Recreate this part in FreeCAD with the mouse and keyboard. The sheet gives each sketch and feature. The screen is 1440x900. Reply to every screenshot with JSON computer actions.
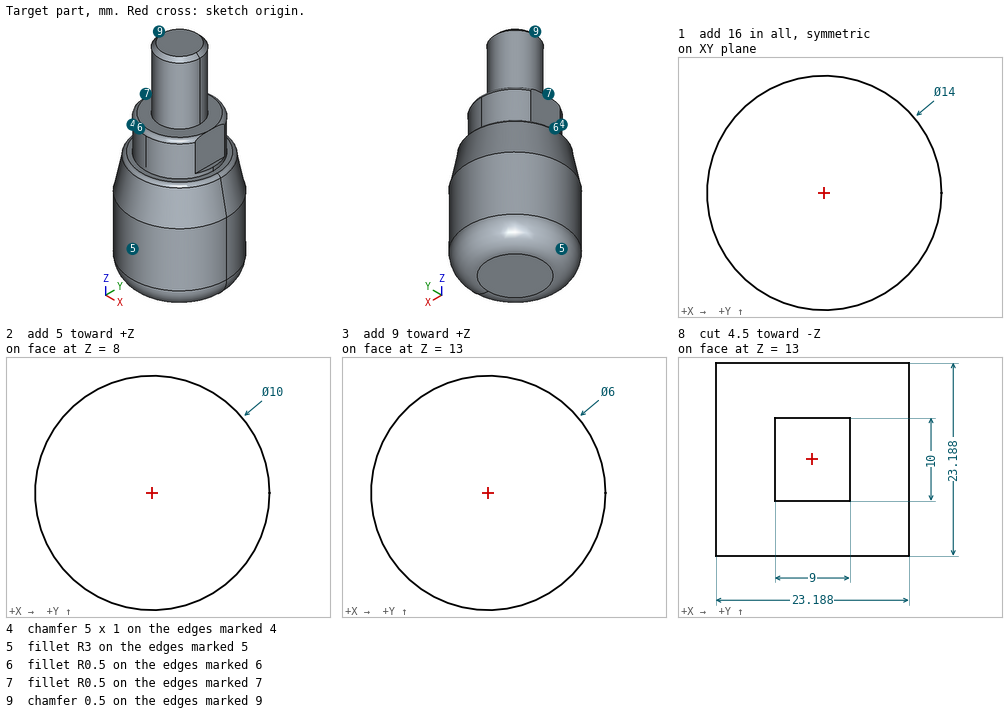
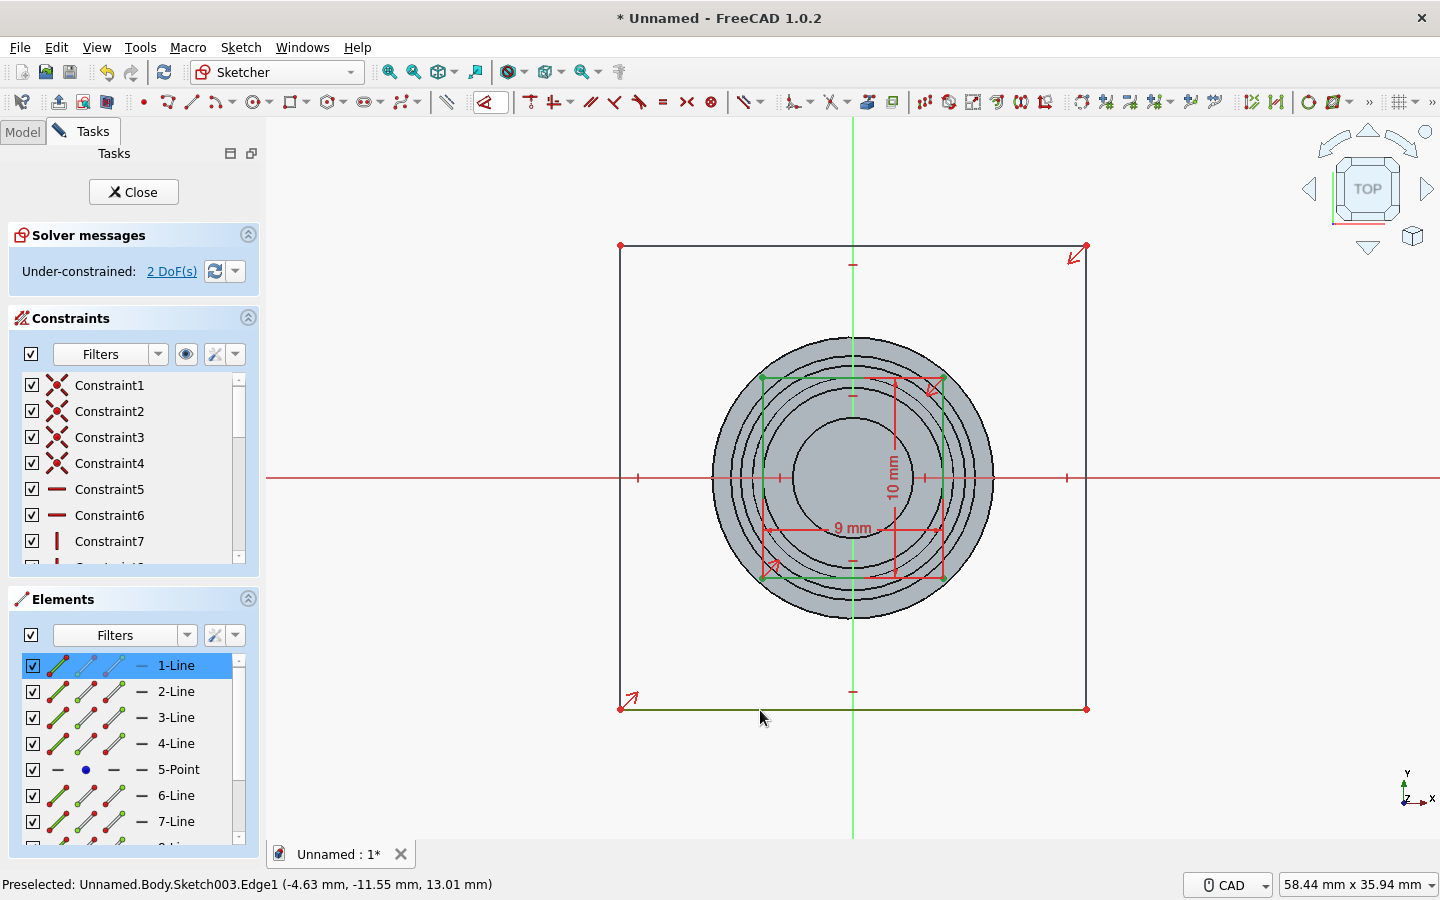
{"action": "key", "text": "l"}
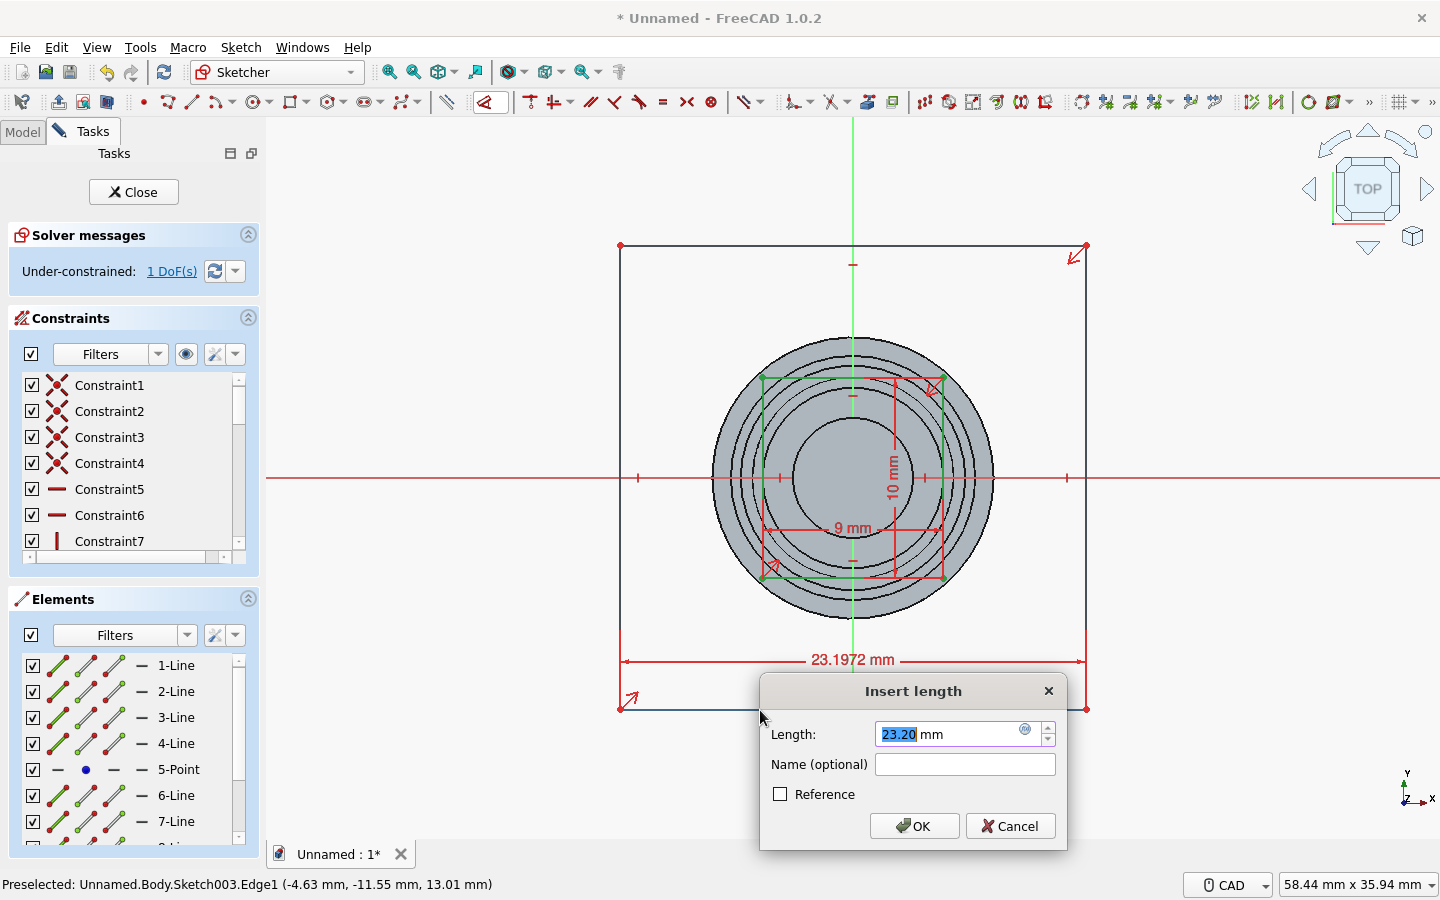
{"action": "type", "text": "23.188"}
{"action": "key", "text": "Return"}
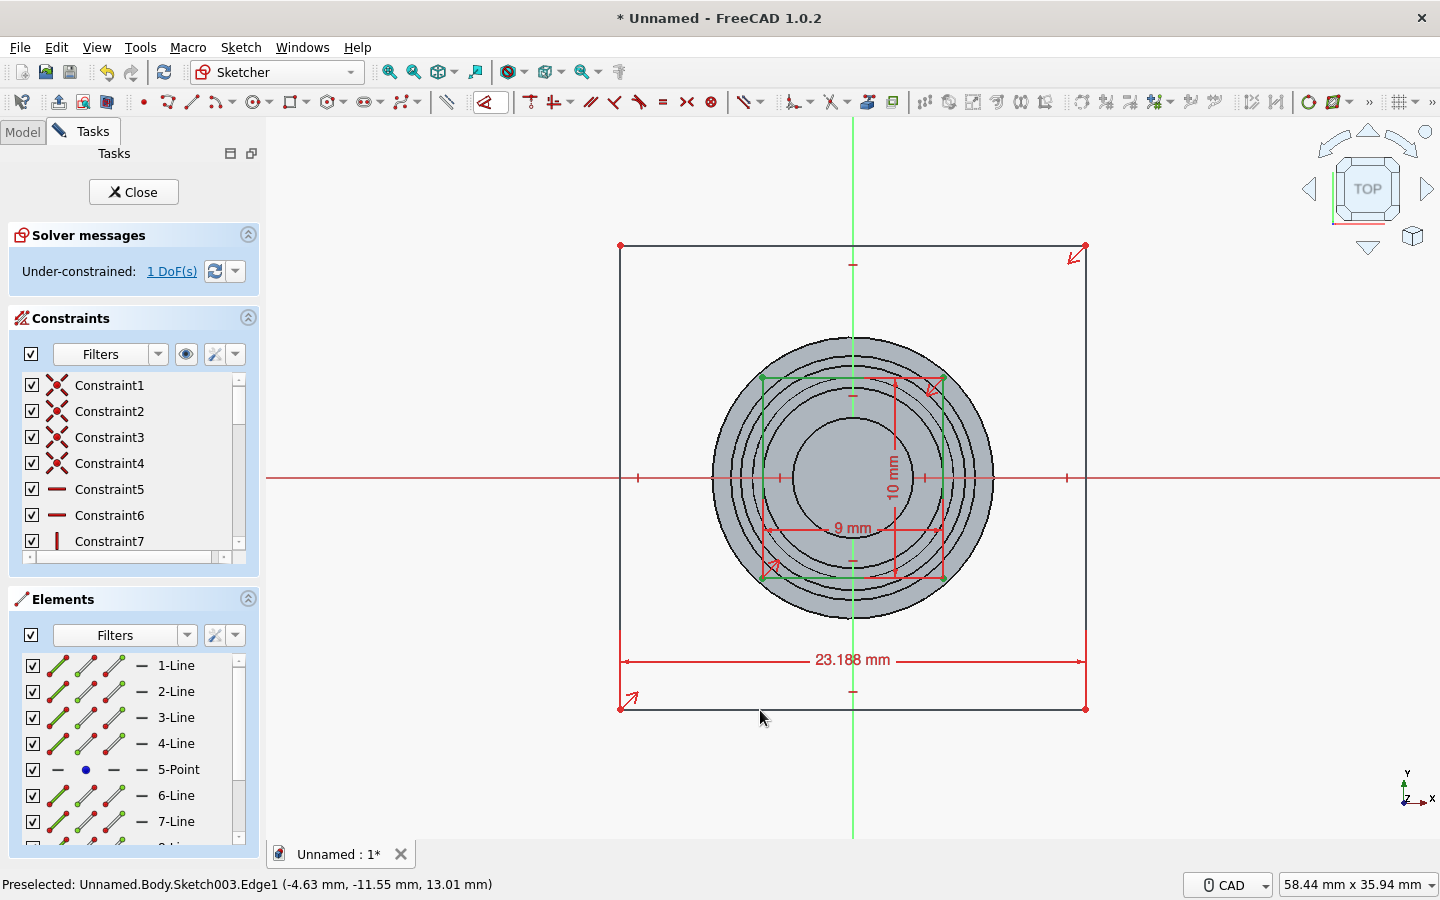
{"action": "left_click", "coordinate": [1086, 571]}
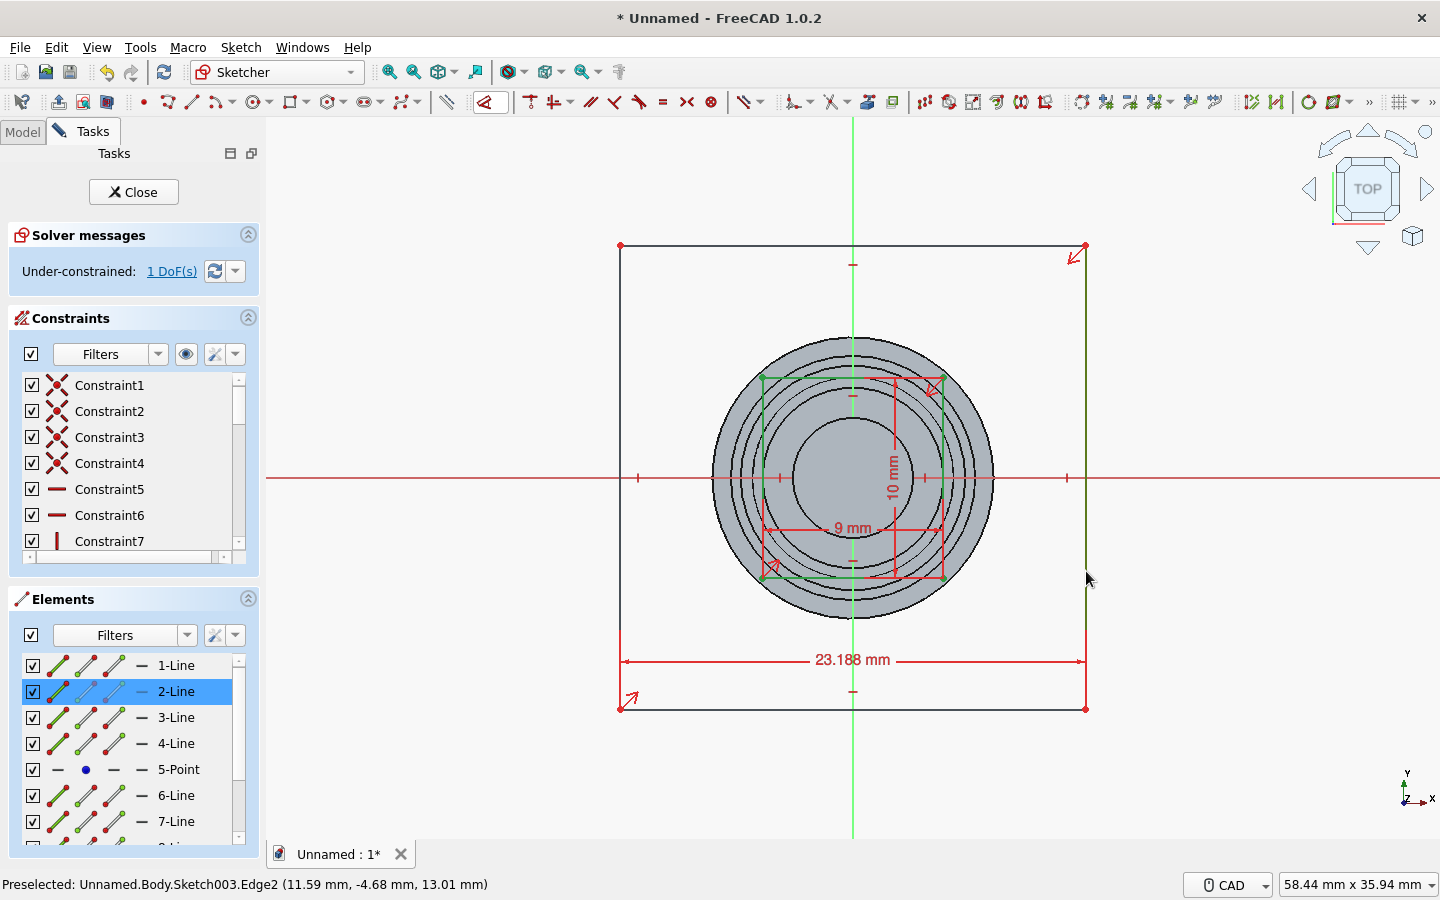
{"action": "key", "text": "i"}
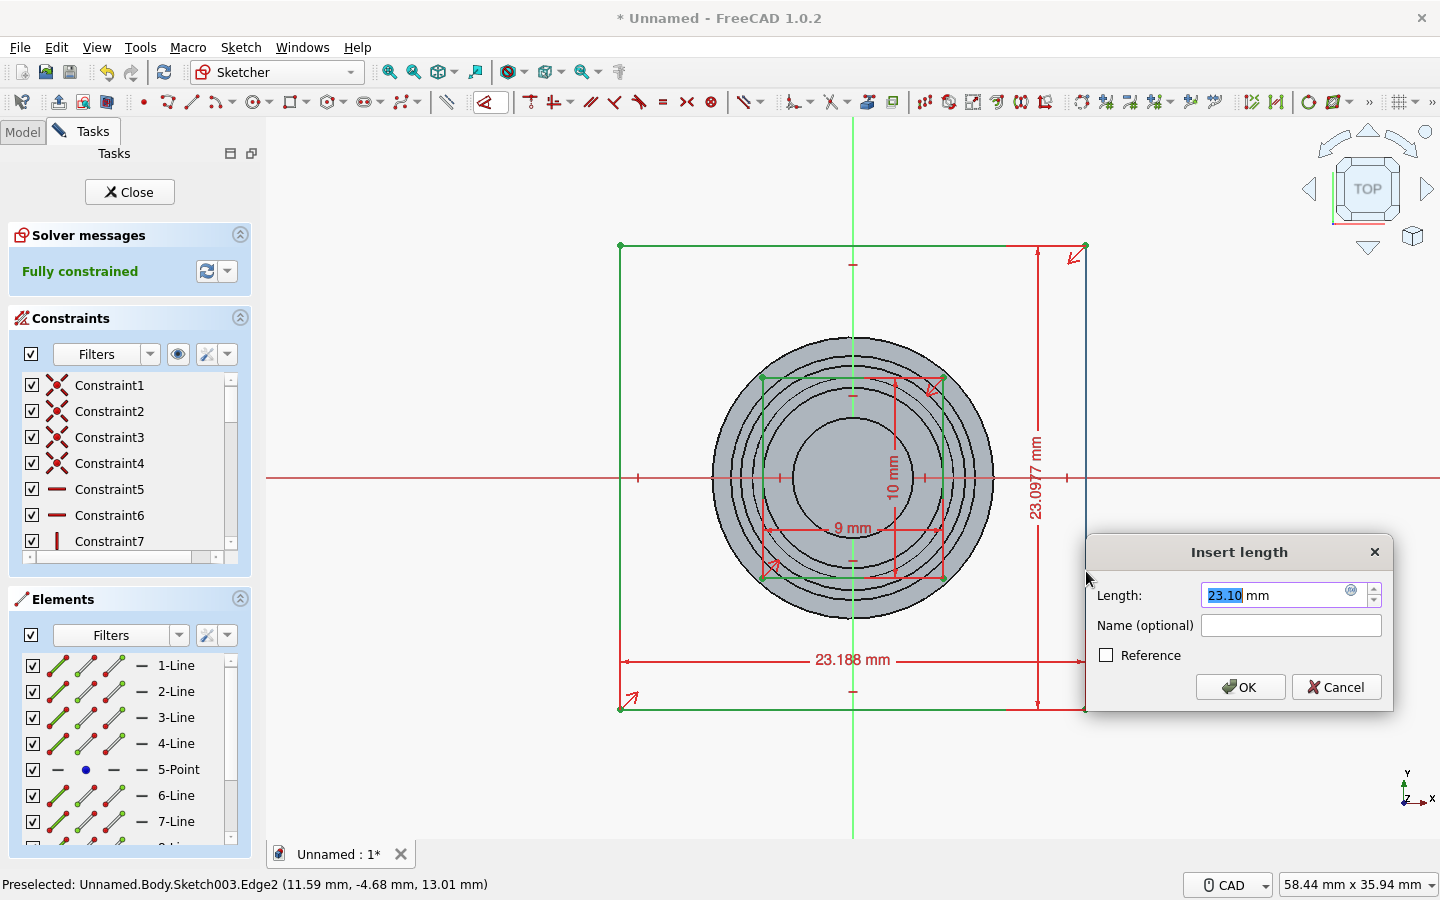
{"action": "type", "text": "23.188"}
{"action": "key", "text": "Return"}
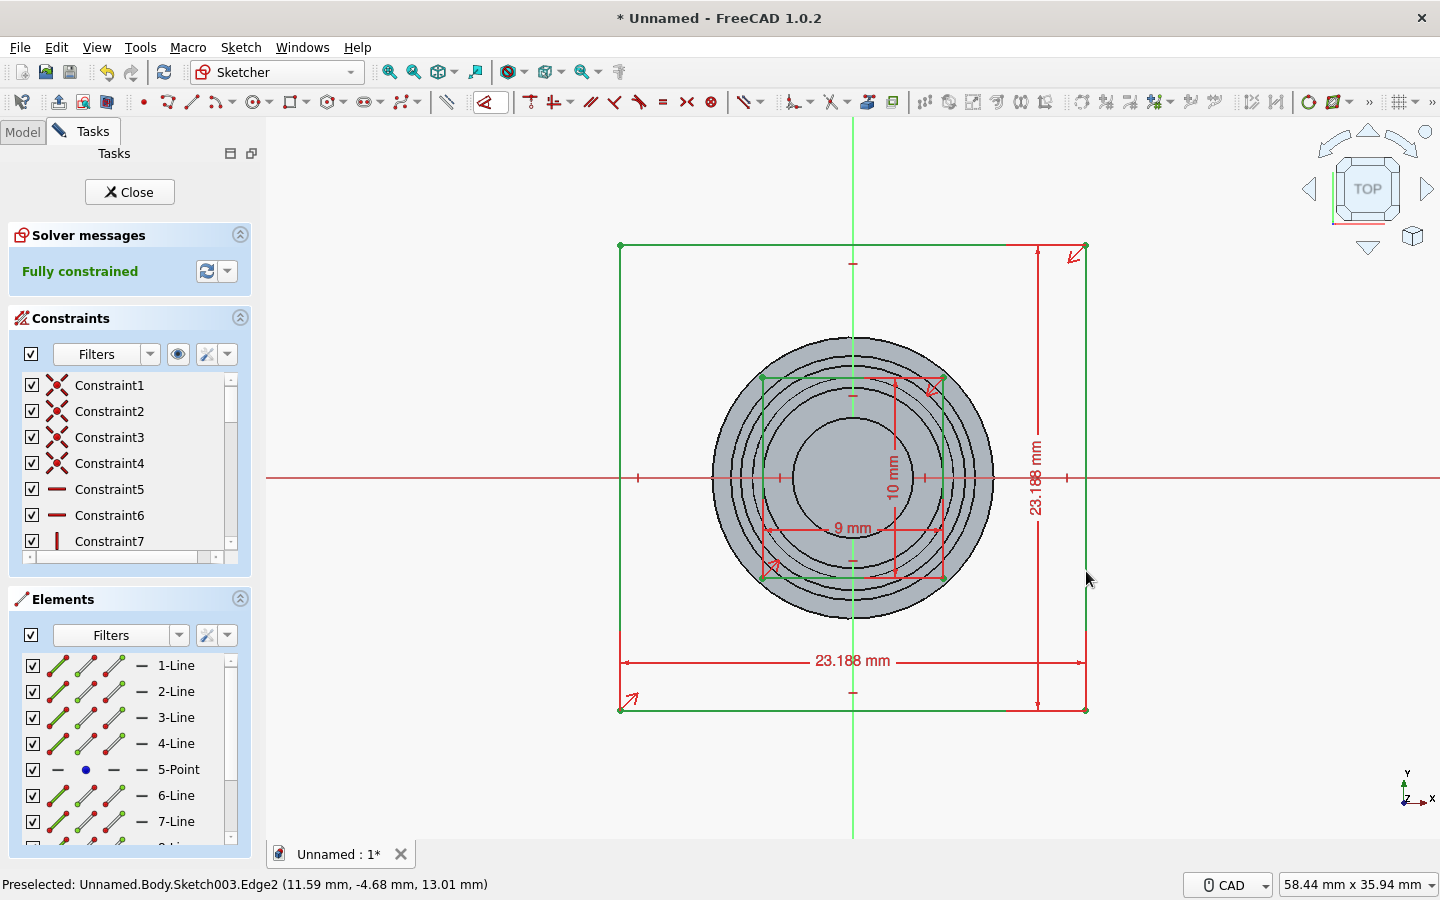
{"action": "left_click", "coordinate": [130, 192]}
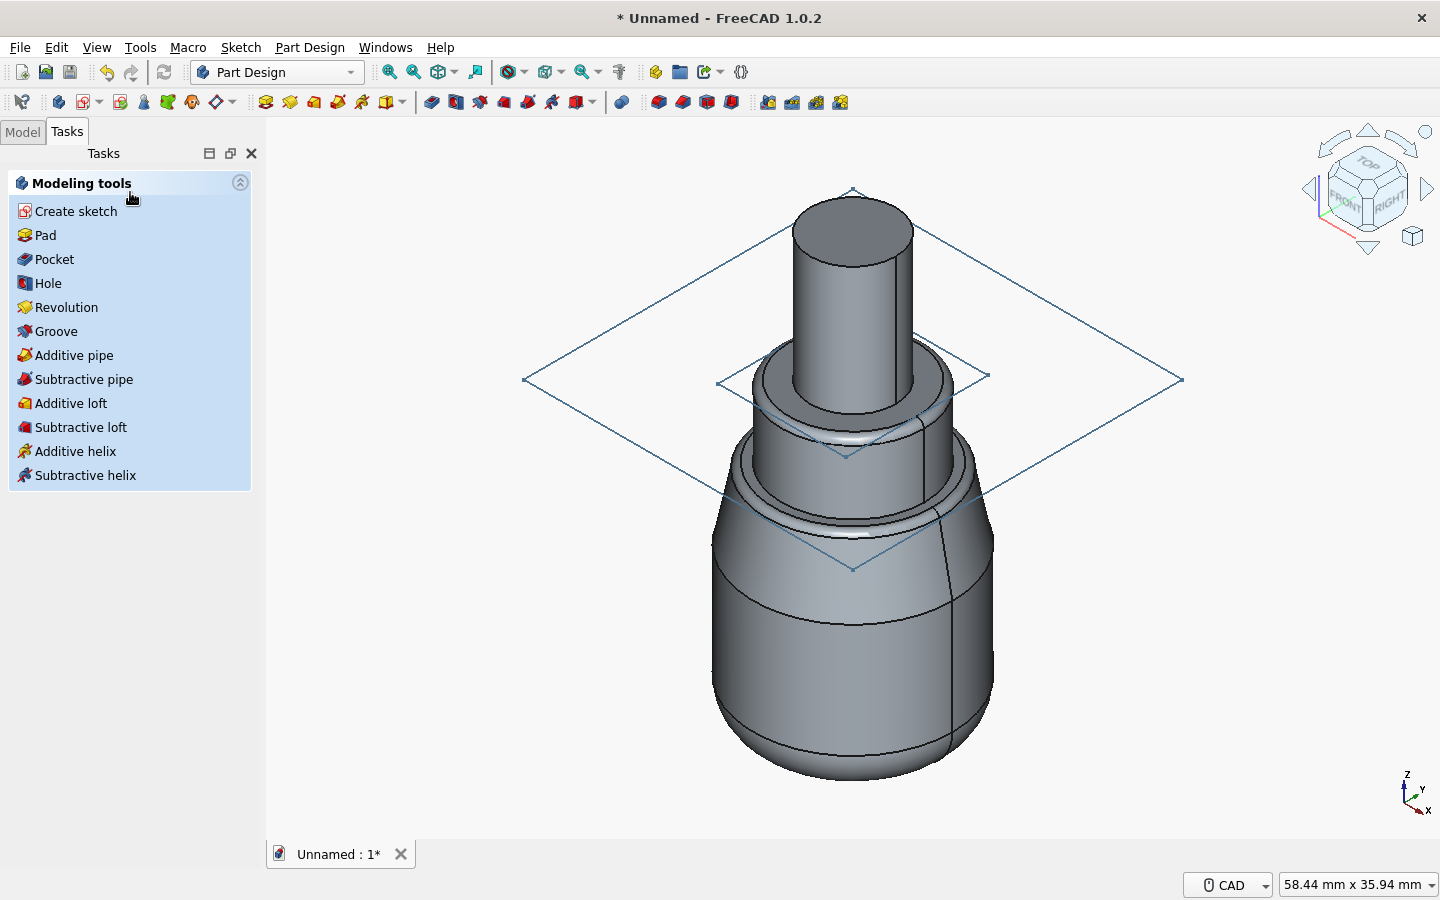
{"action": "left_click", "coordinate": [432, 102]}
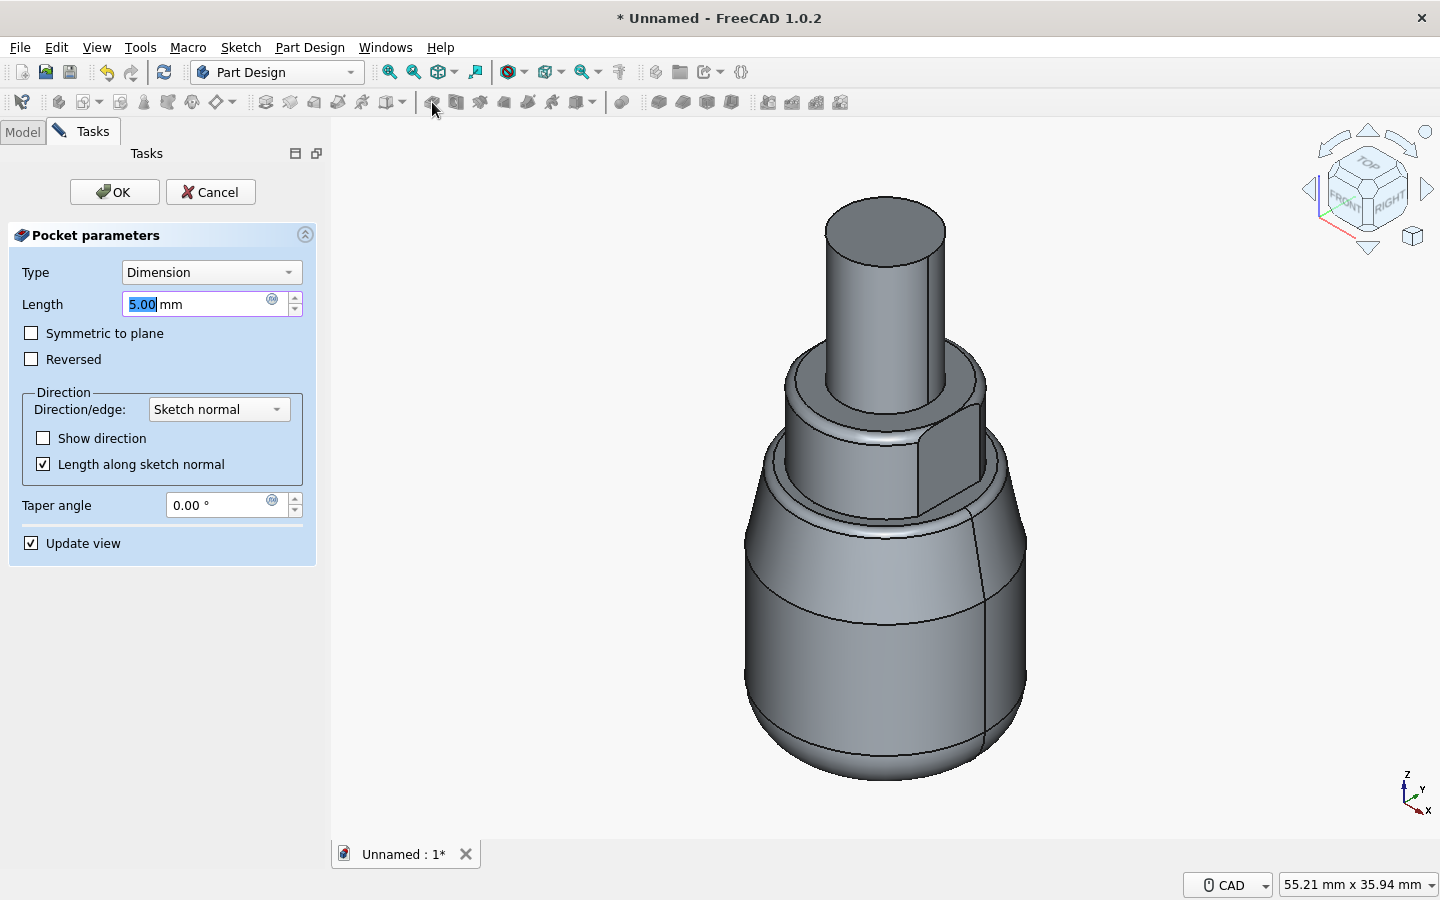
{"action": "type", "text": "4.5"}
{"action": "key", "text": "Tab"}